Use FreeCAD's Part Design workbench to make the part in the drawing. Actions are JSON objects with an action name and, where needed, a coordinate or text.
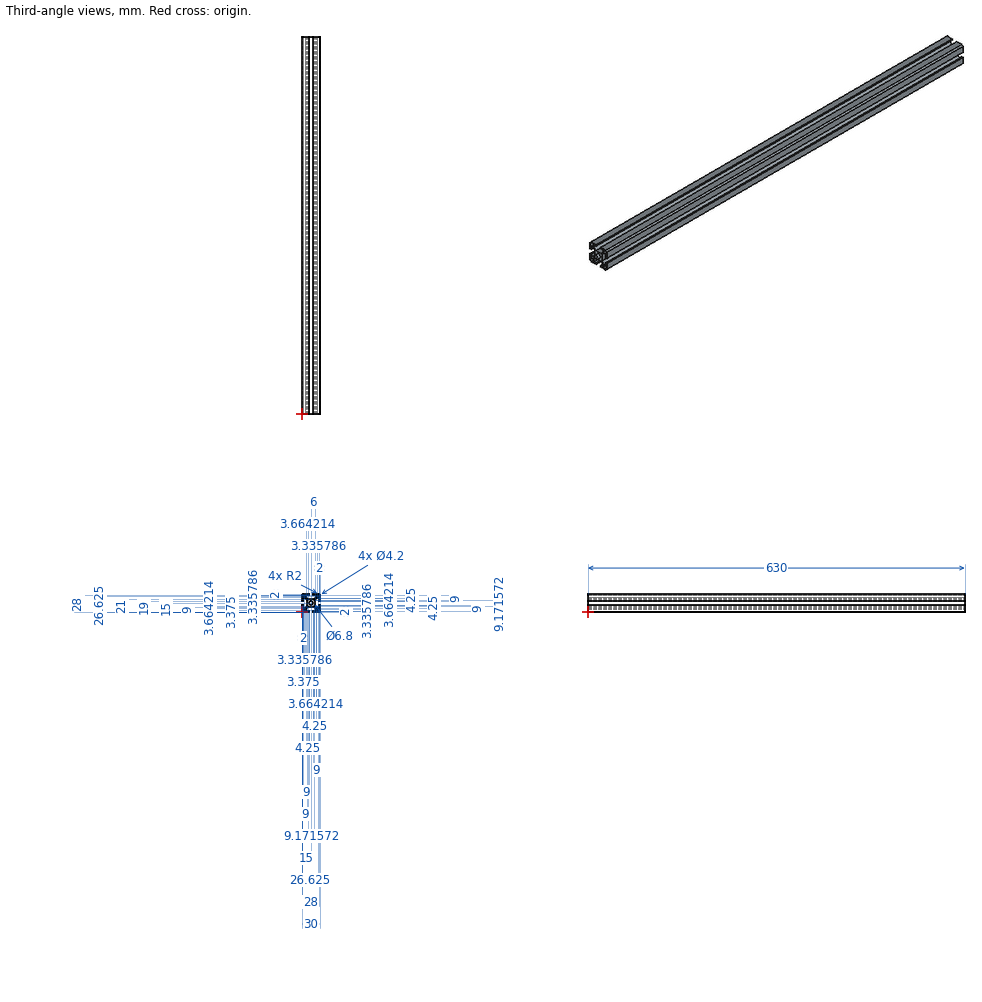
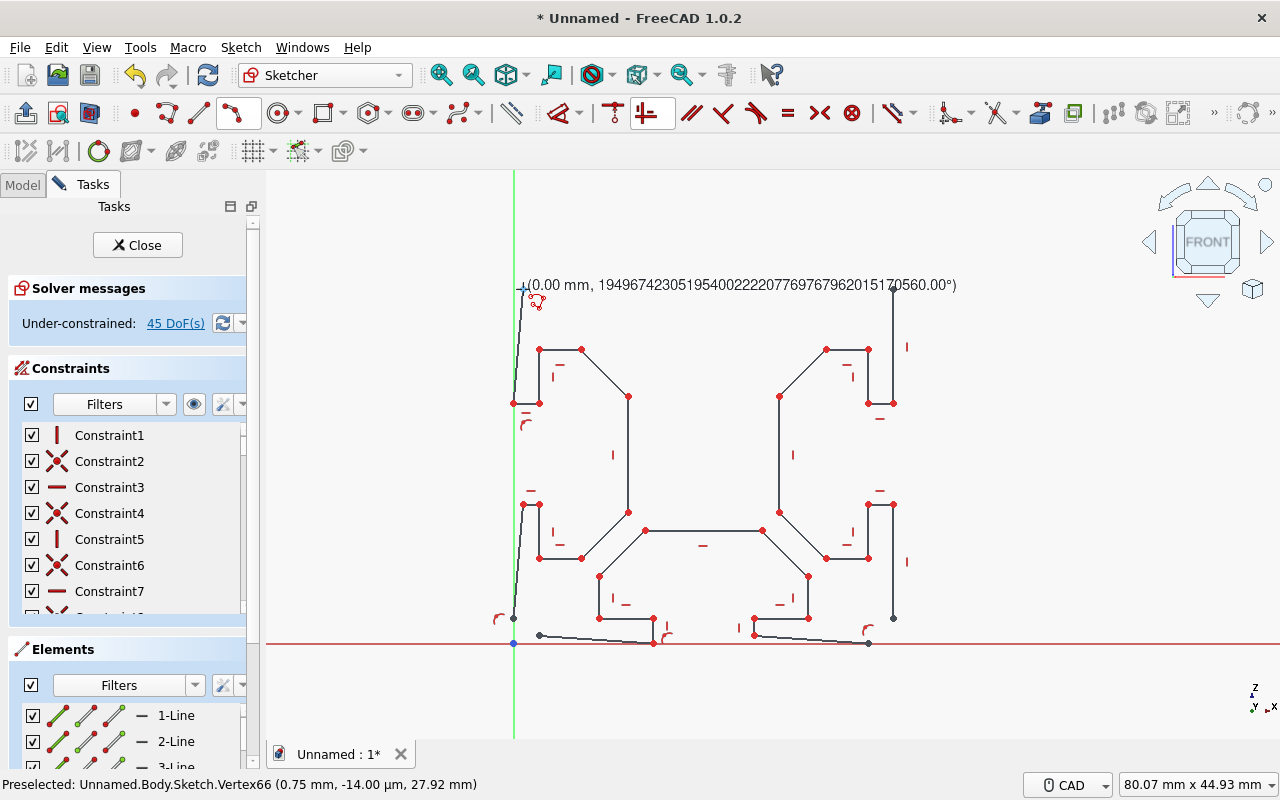
{"action": "left_click", "coordinate": [539, 264]}
{"action": "left_click", "coordinate": [653, 264]}
{"action": "left_click", "coordinate": [653, 289]}
{"action": "left_click", "coordinate": [599, 289]}
{"action": "left_click", "coordinate": [599, 331]}
{"action": "left_click", "coordinate": [645, 378]}
{"action": "left_click", "coordinate": [762, 378]}
{"action": "left_click", "coordinate": [808, 331]}
{"action": "left_click", "coordinate": [808, 289]}
{"action": "left_click", "coordinate": [754, 289]}
{"action": "left_click", "coordinate": [754, 264]}
{"action": "left_click", "coordinate": [868, 264]}
{"action": "right_click", "coordinate": [868, 264]}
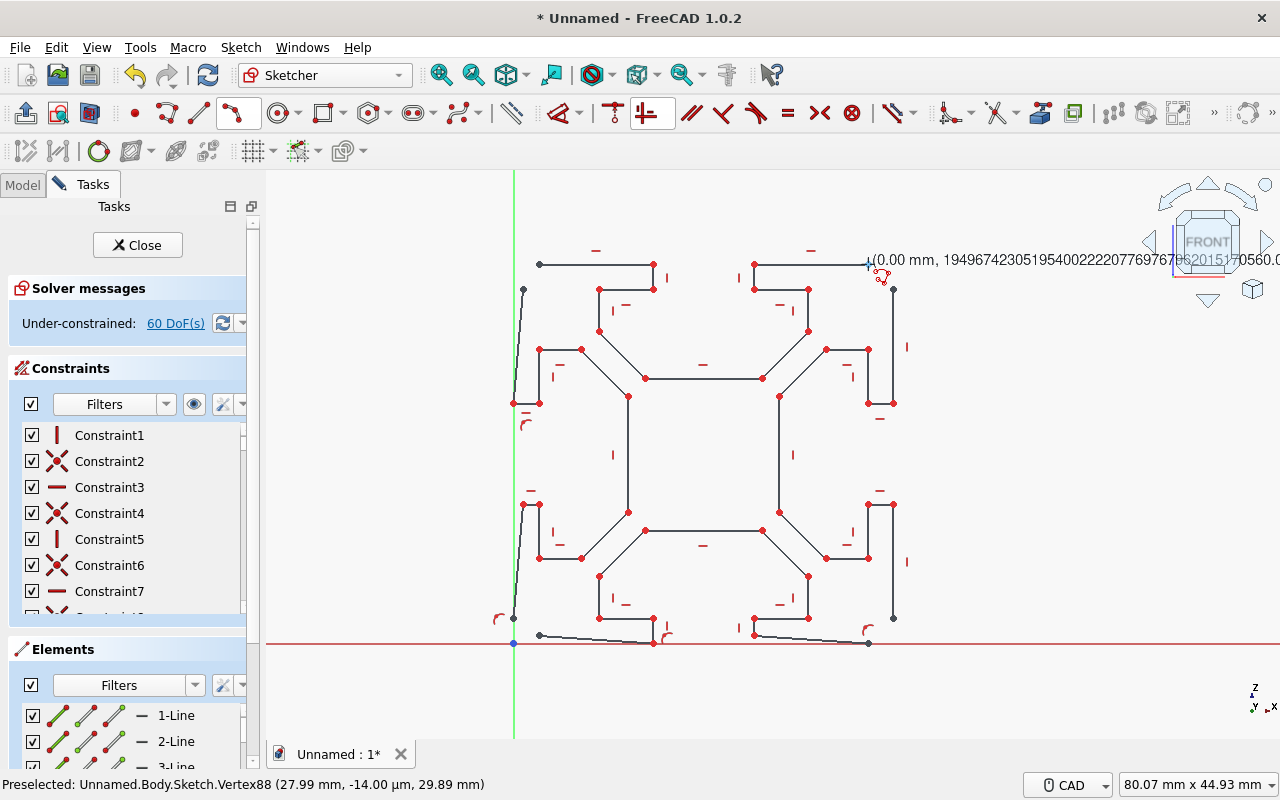
{"action": "left_click", "coordinate": [232, 114]}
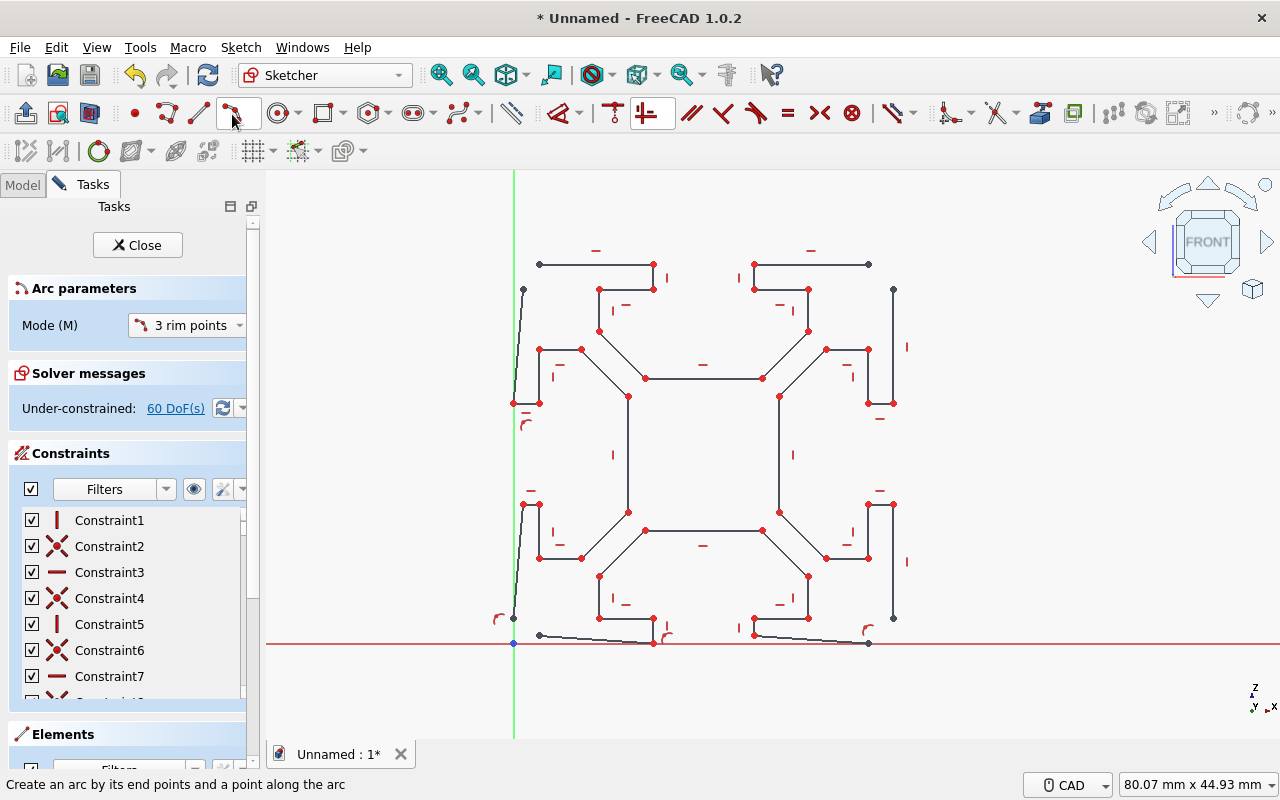
{"action": "left_click", "coordinate": [893, 619]}
{"action": "left_click", "coordinate": [868, 644]}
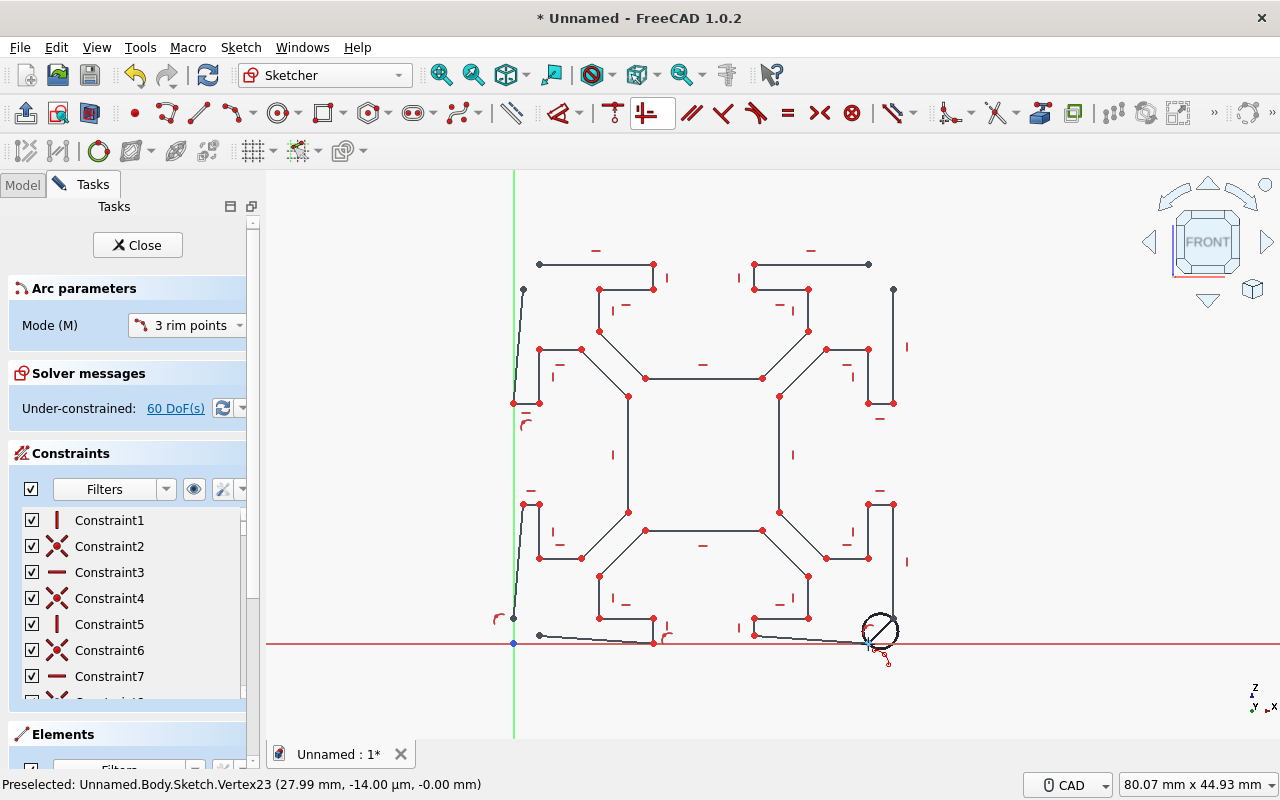
{"action": "scroll", "coordinate": [886, 636], "scroll_direction": "up", "scroll_amount": 4}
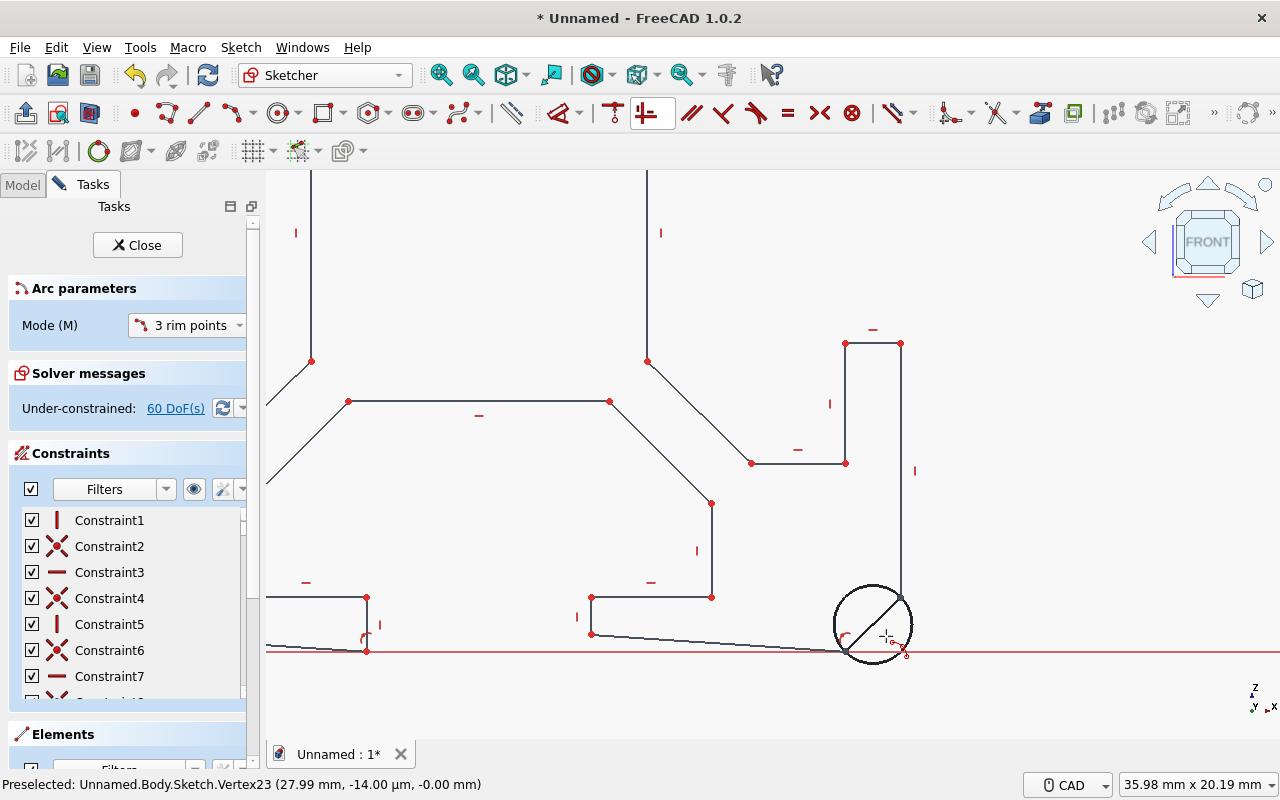
{"action": "left_click", "coordinate": [885, 635]}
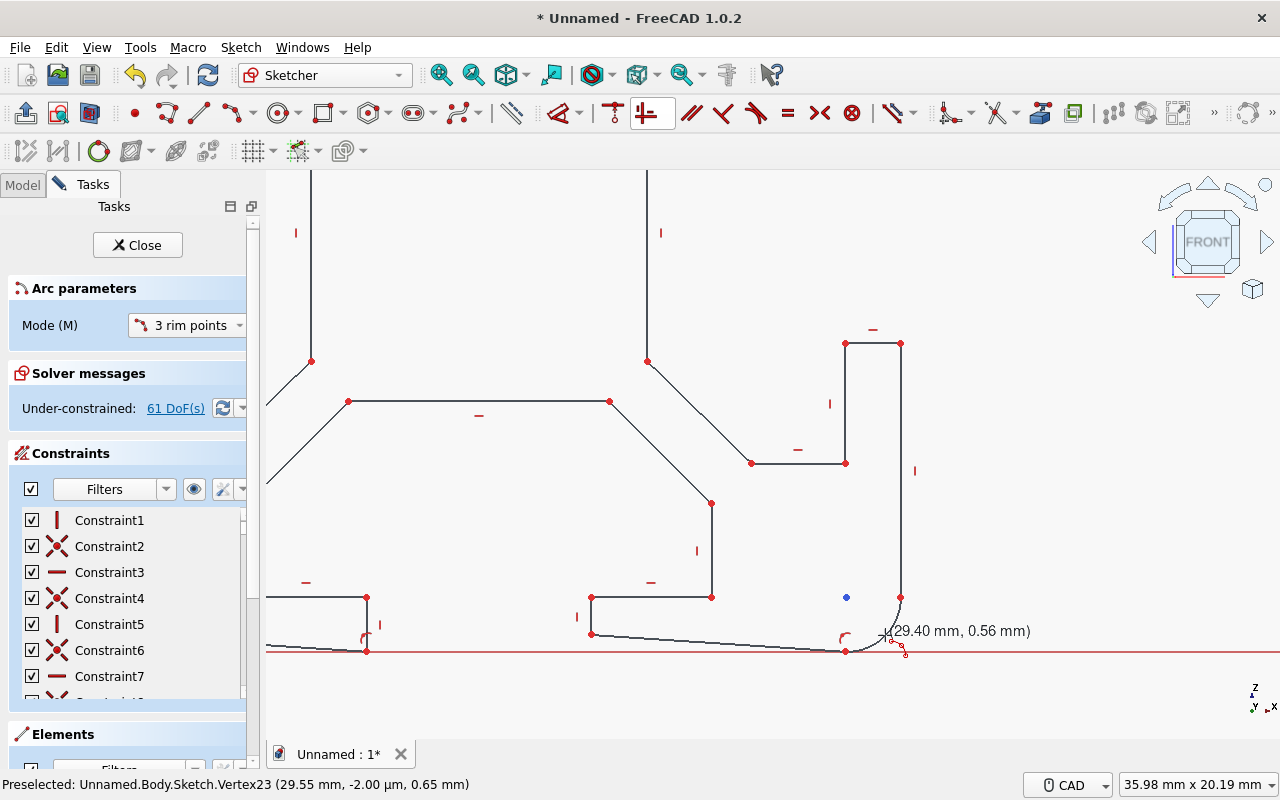
{"action": "scroll", "coordinate": [888, 638], "scroll_direction": "down", "scroll_amount": 4}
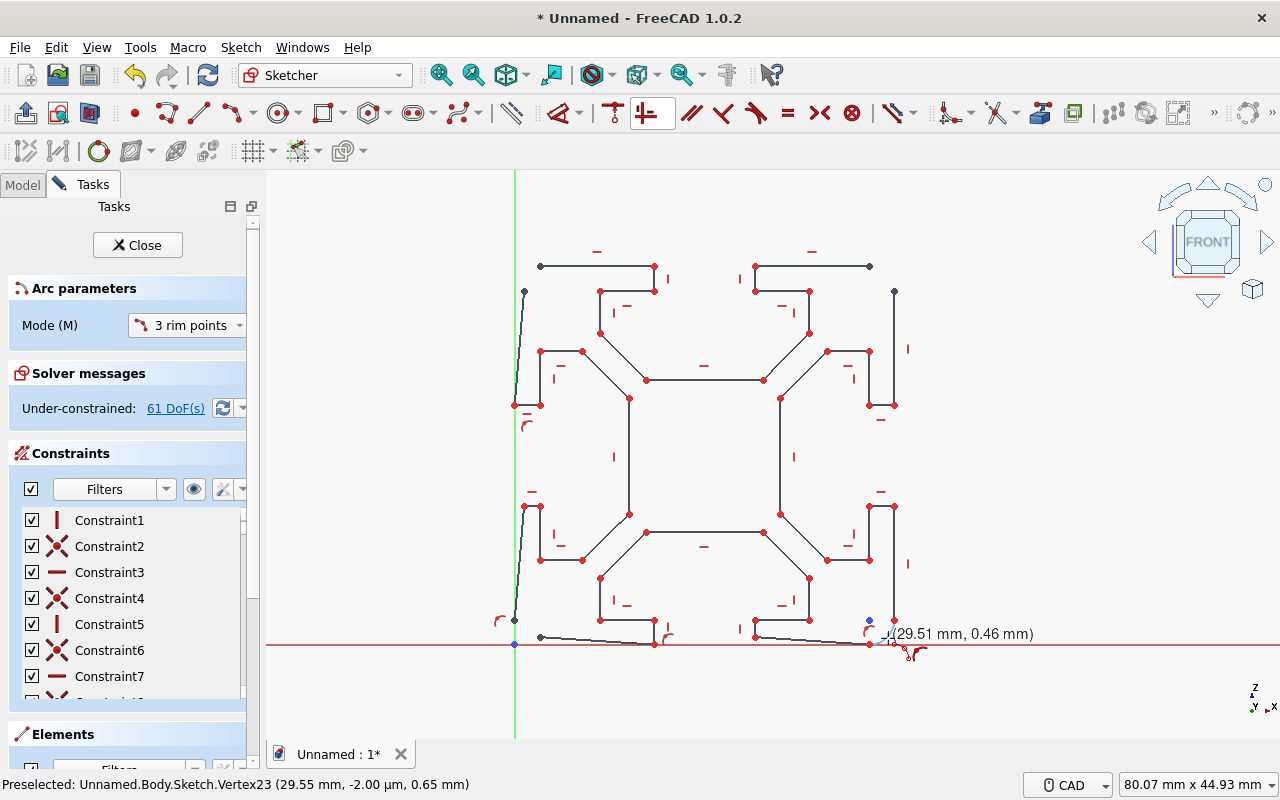
{"action": "left_click", "coordinate": [540, 637]}
{"action": "left_click", "coordinate": [515, 620]}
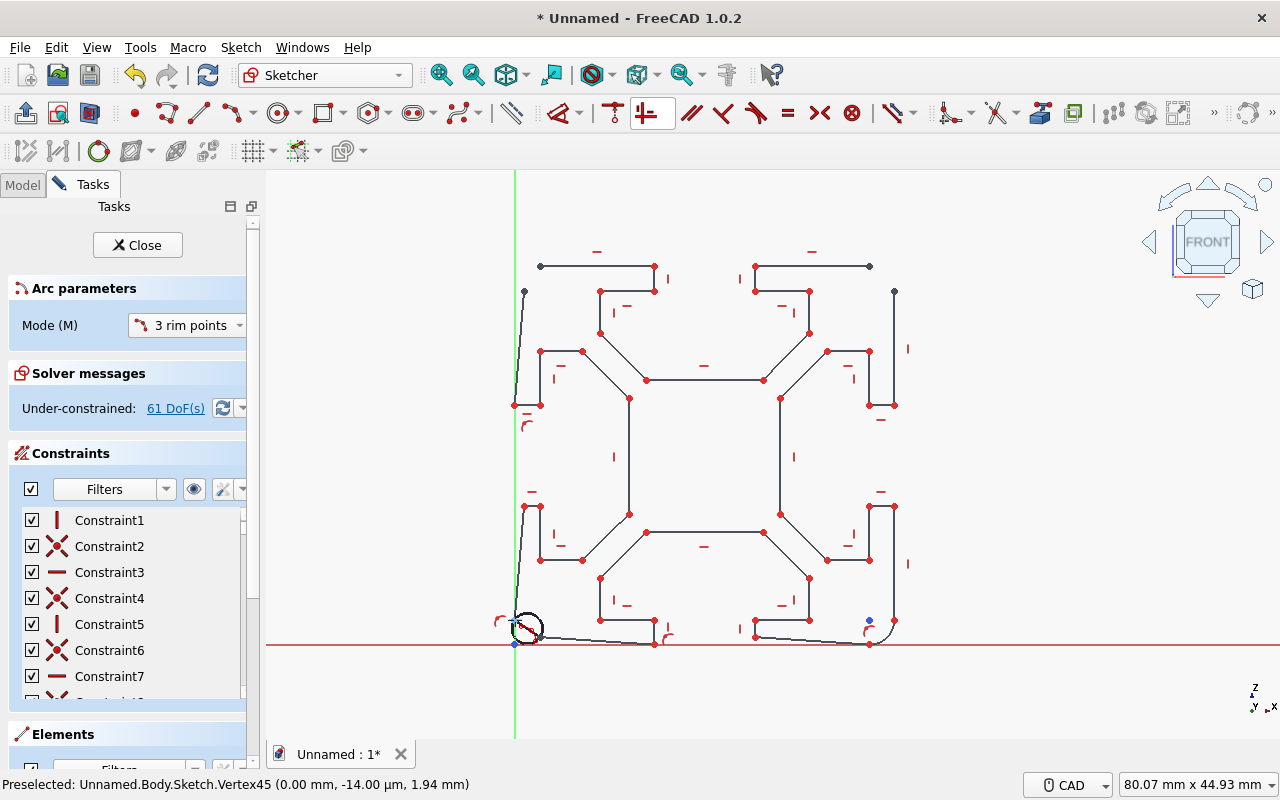
{"action": "scroll", "coordinate": [522, 637], "scroll_direction": "up", "scroll_amount": 4}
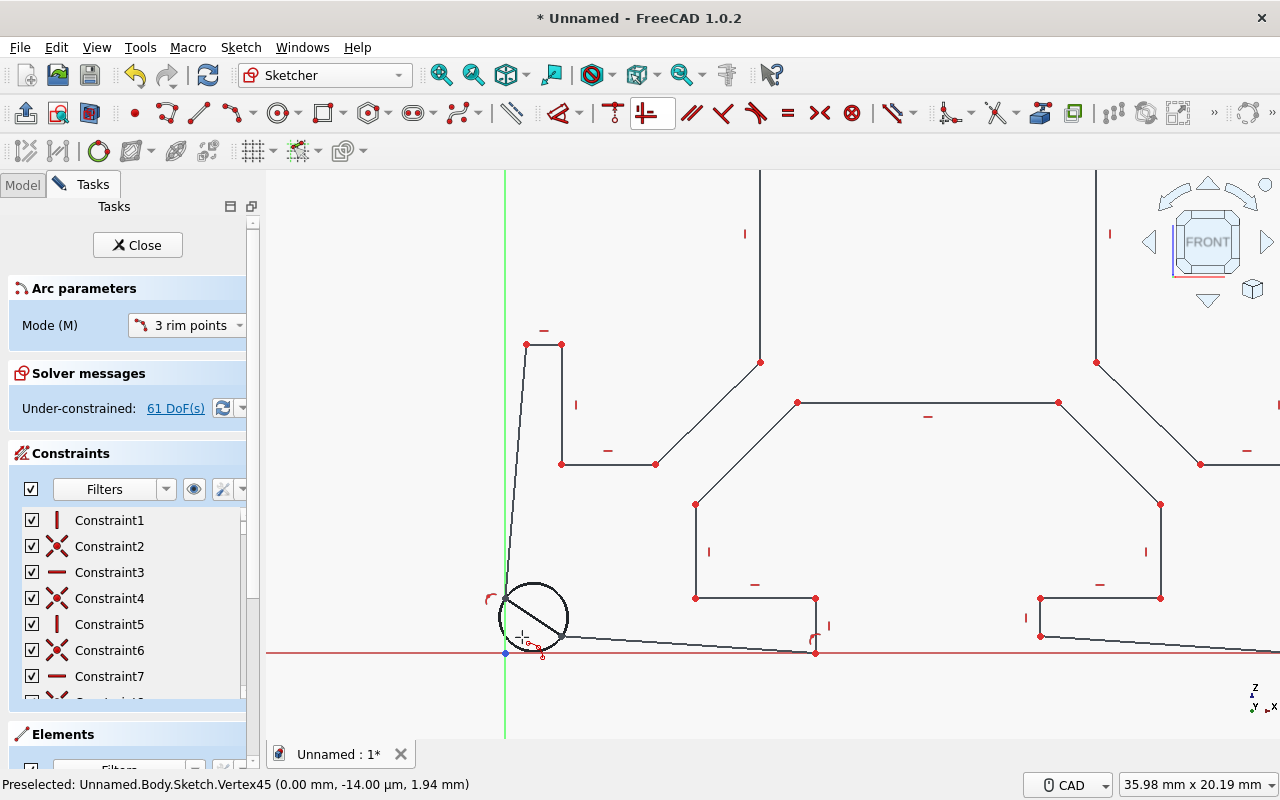
{"action": "left_click", "coordinate": [522, 637]}